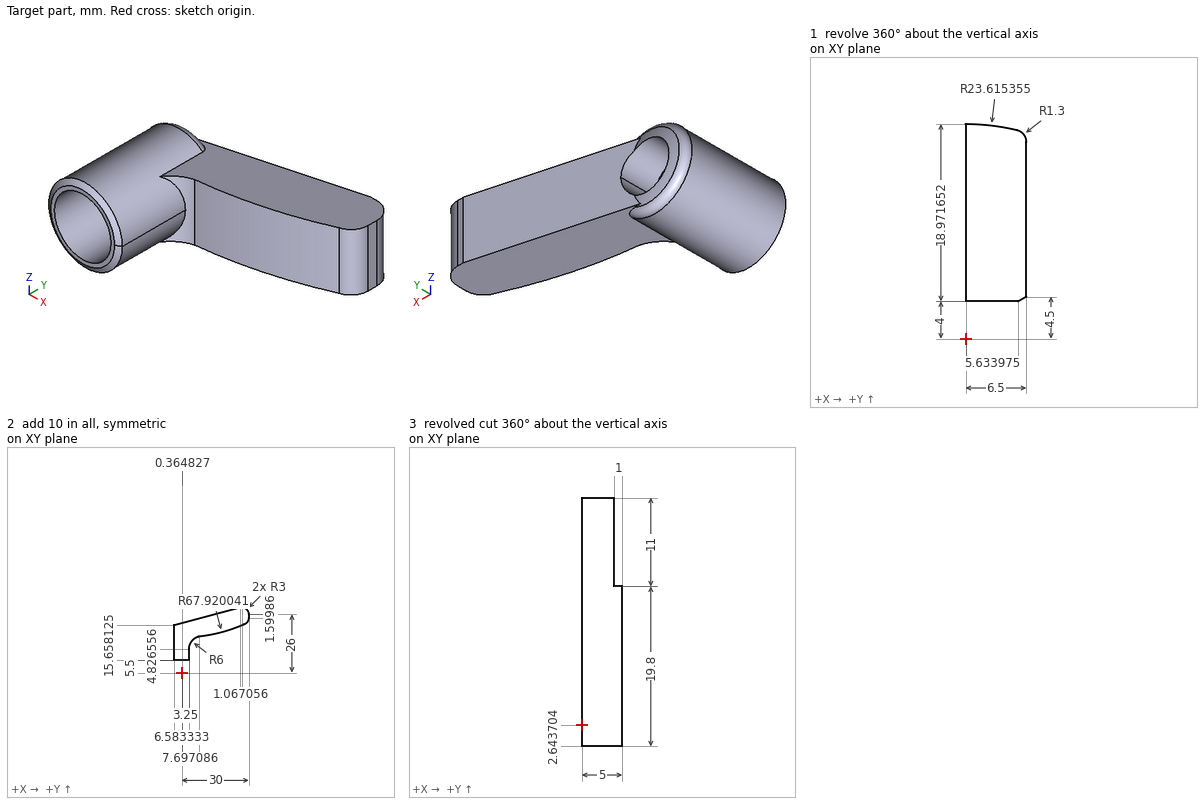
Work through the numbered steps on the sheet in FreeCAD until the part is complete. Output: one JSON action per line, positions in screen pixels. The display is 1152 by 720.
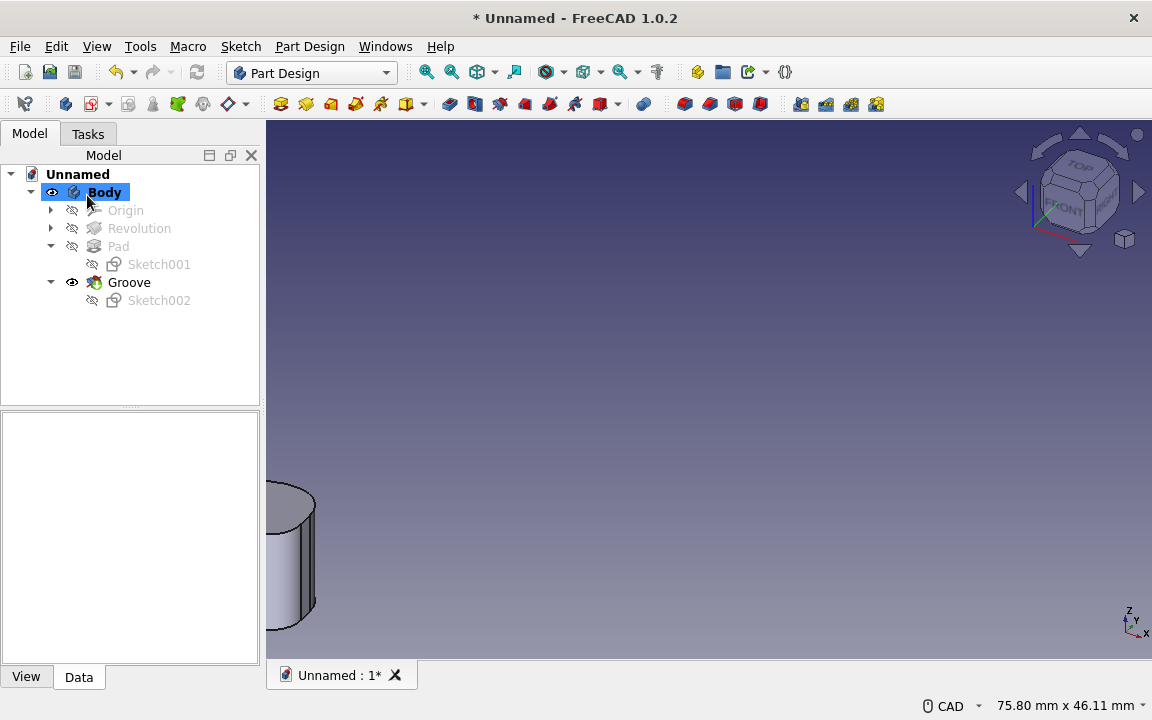
{"action": "key", "text": "0"}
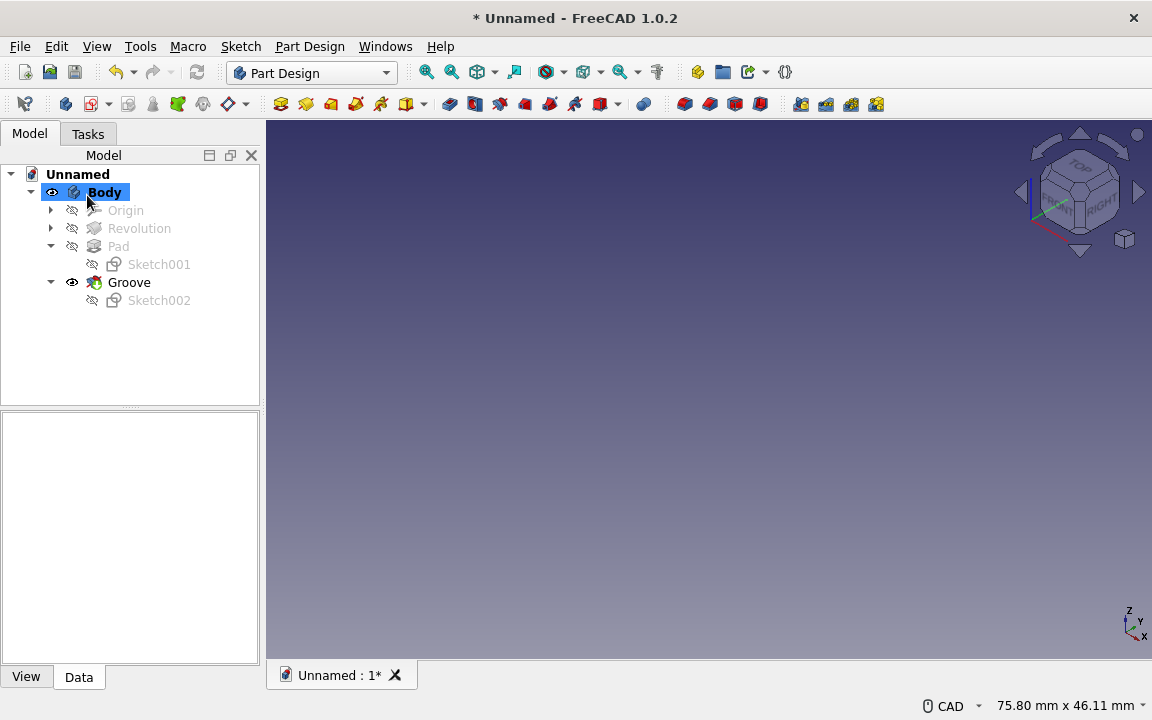
{"action": "key", "text": "v f"}